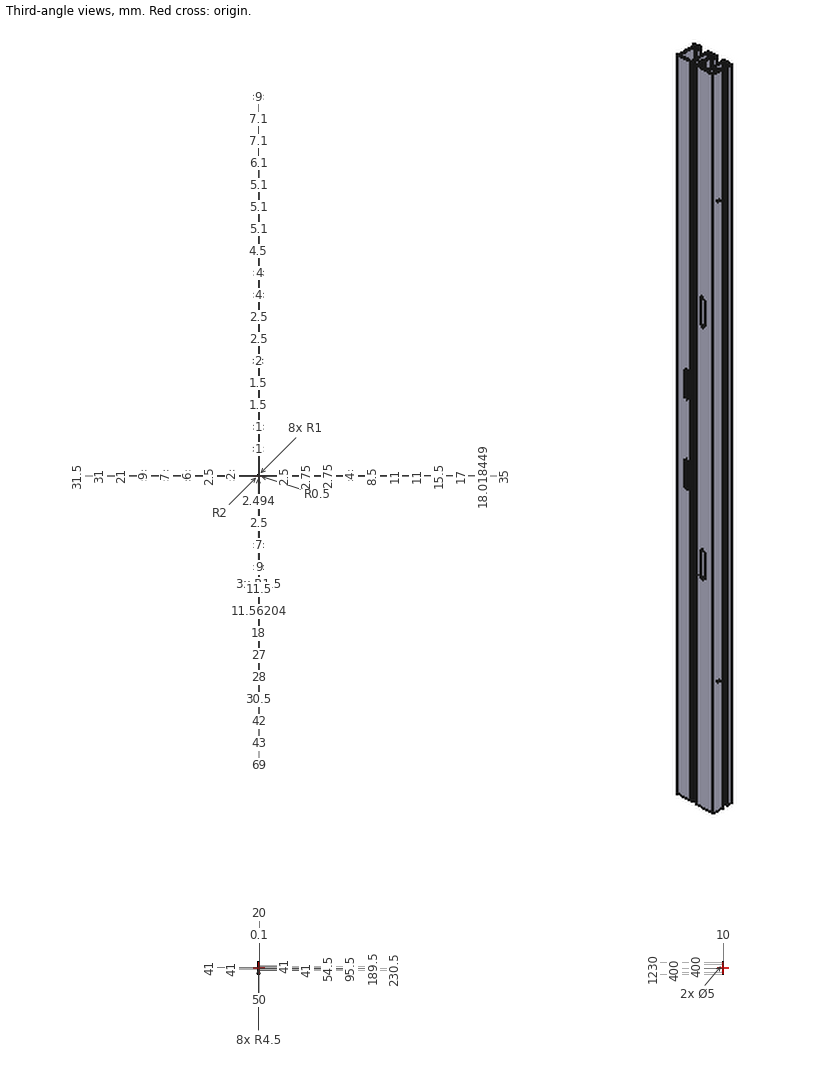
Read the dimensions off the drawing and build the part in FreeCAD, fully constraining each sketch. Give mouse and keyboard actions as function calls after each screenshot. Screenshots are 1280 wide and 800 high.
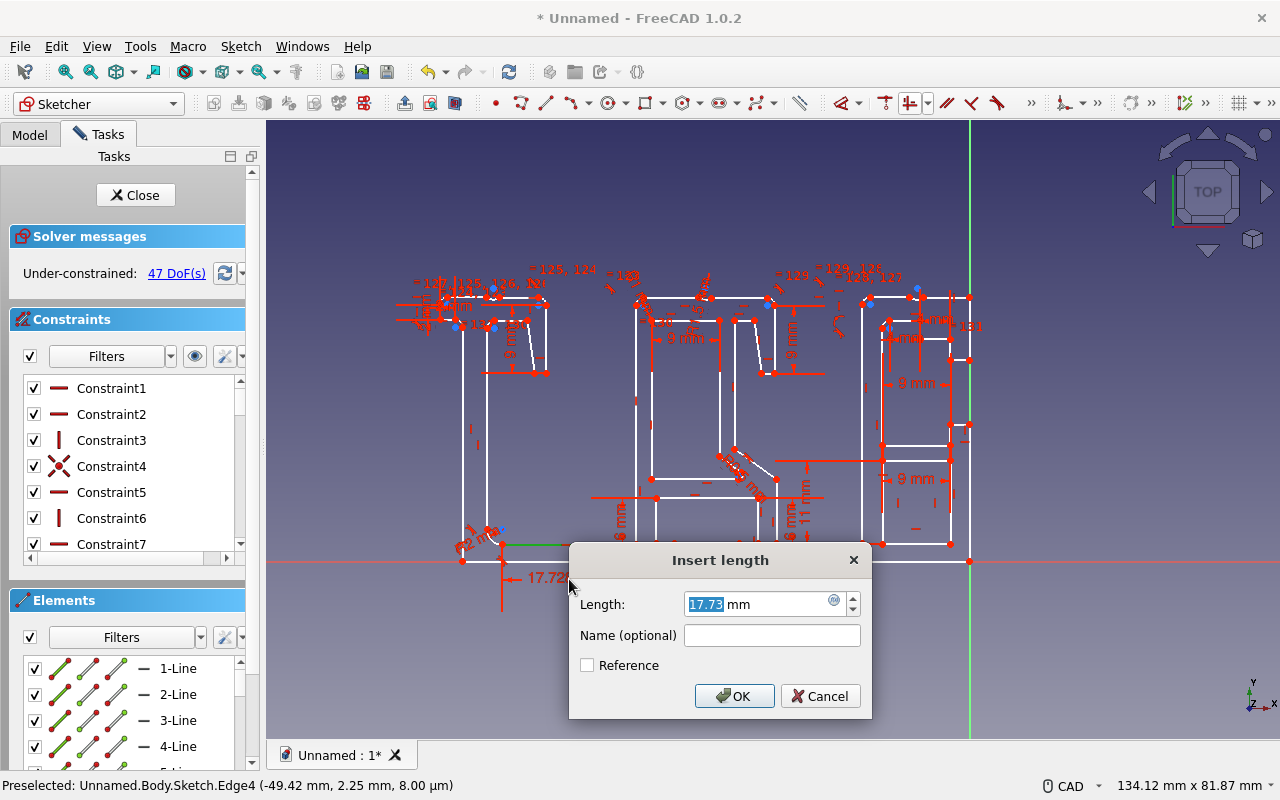
text(18)
key(Return)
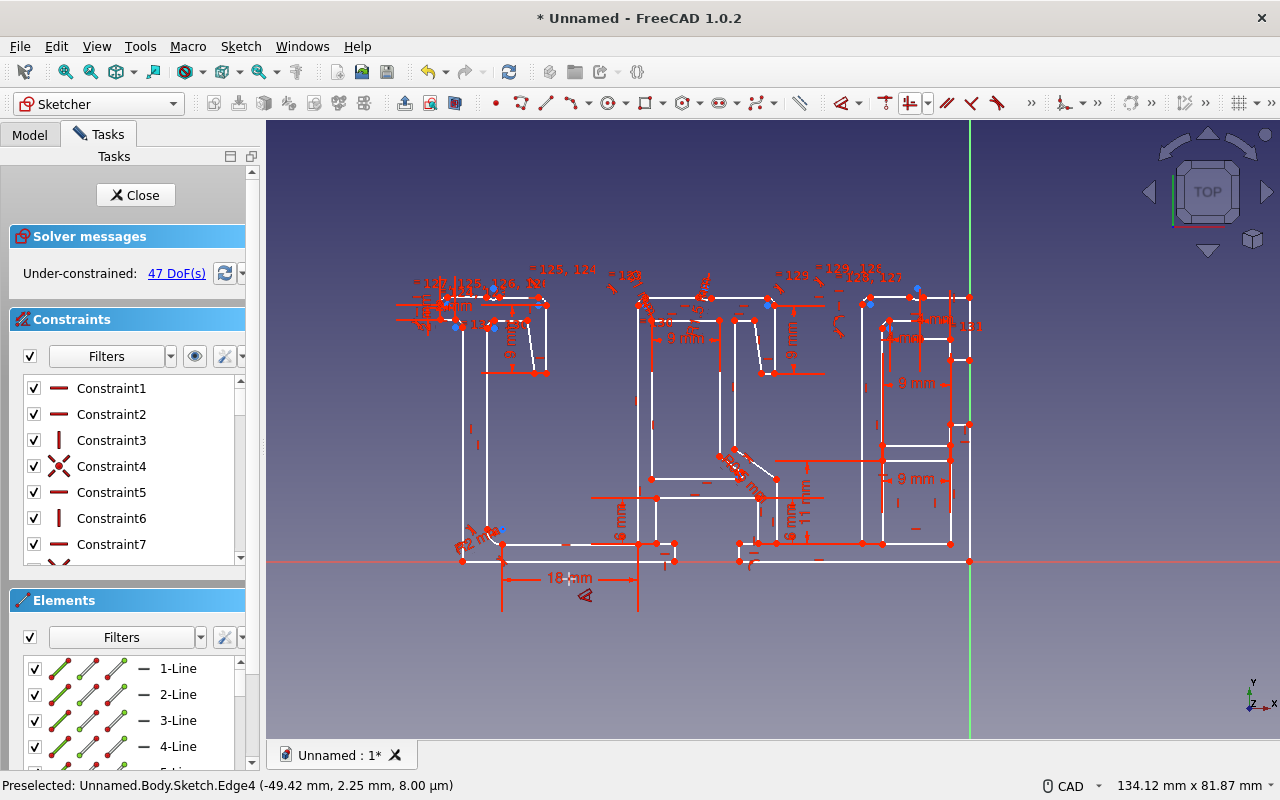
click(463, 398)
click(429, 445)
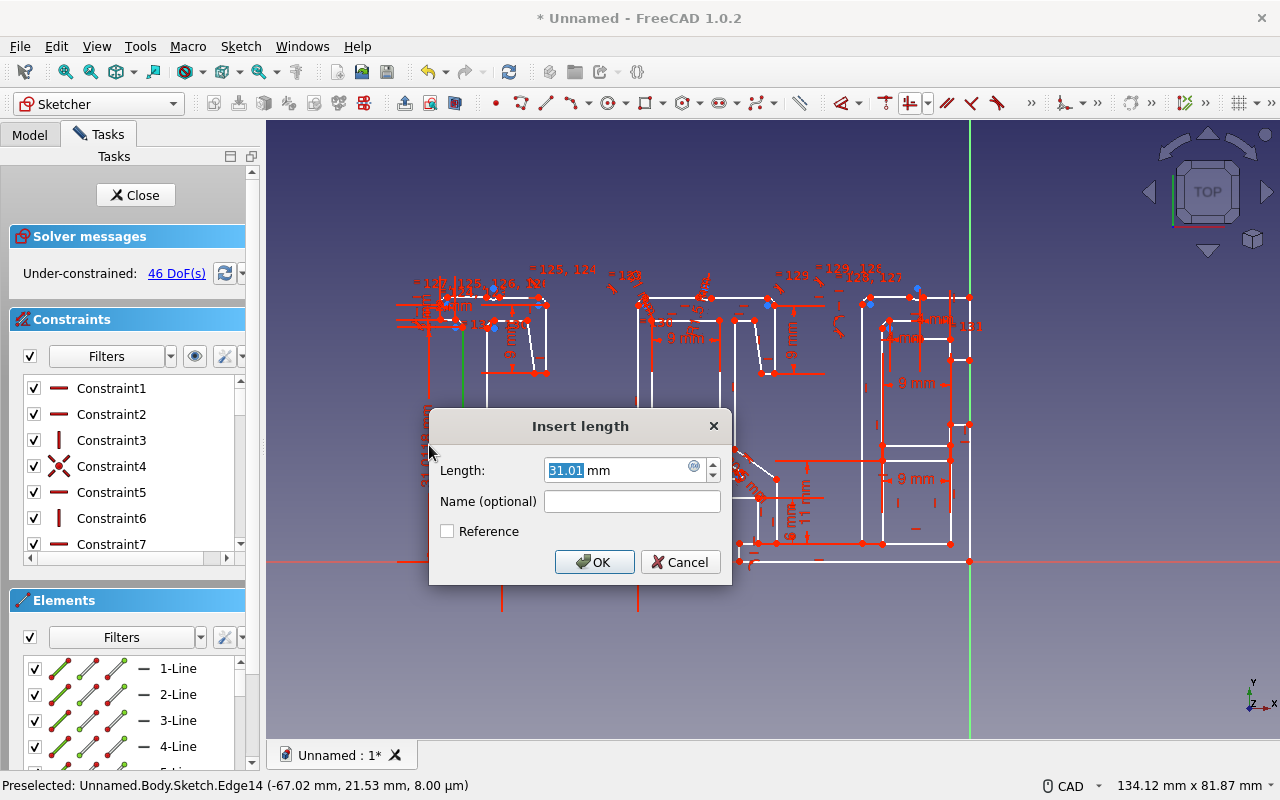
text(31)
key(Return)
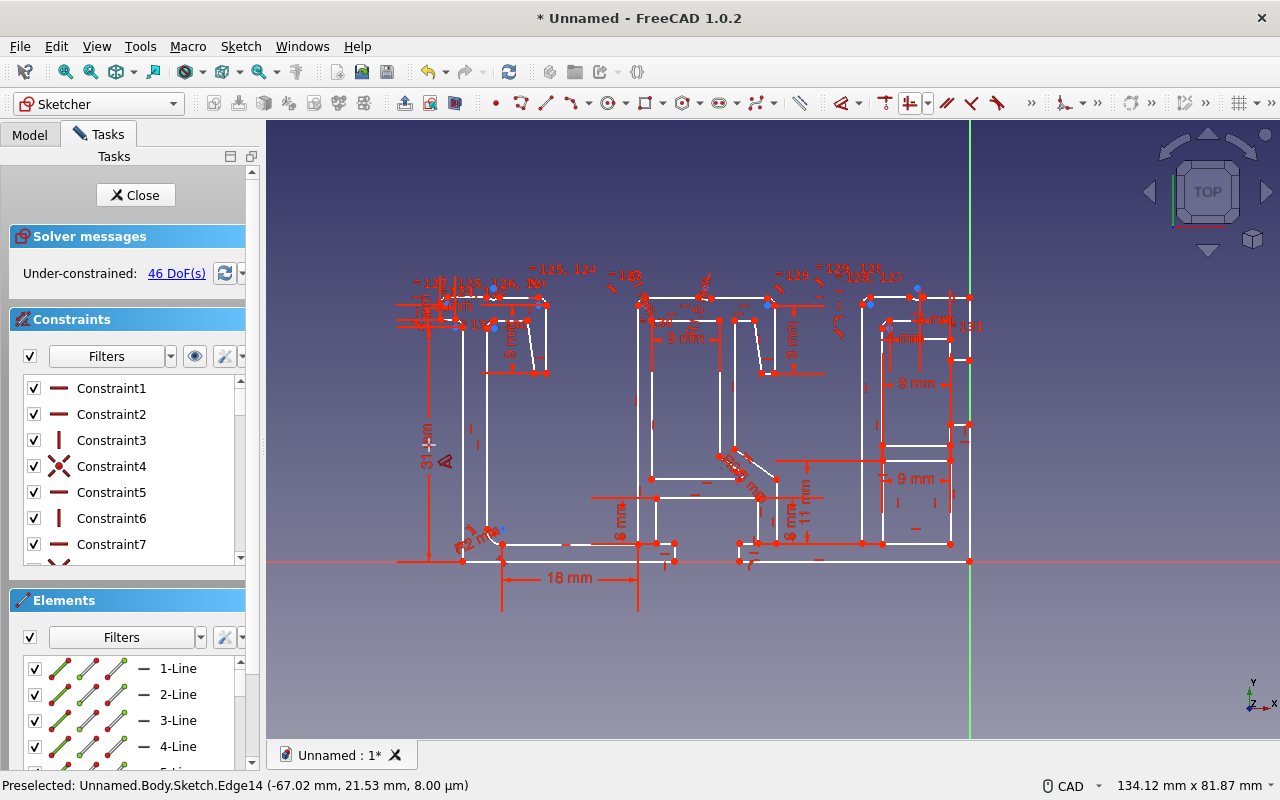
click(526, 562)
click(495, 596)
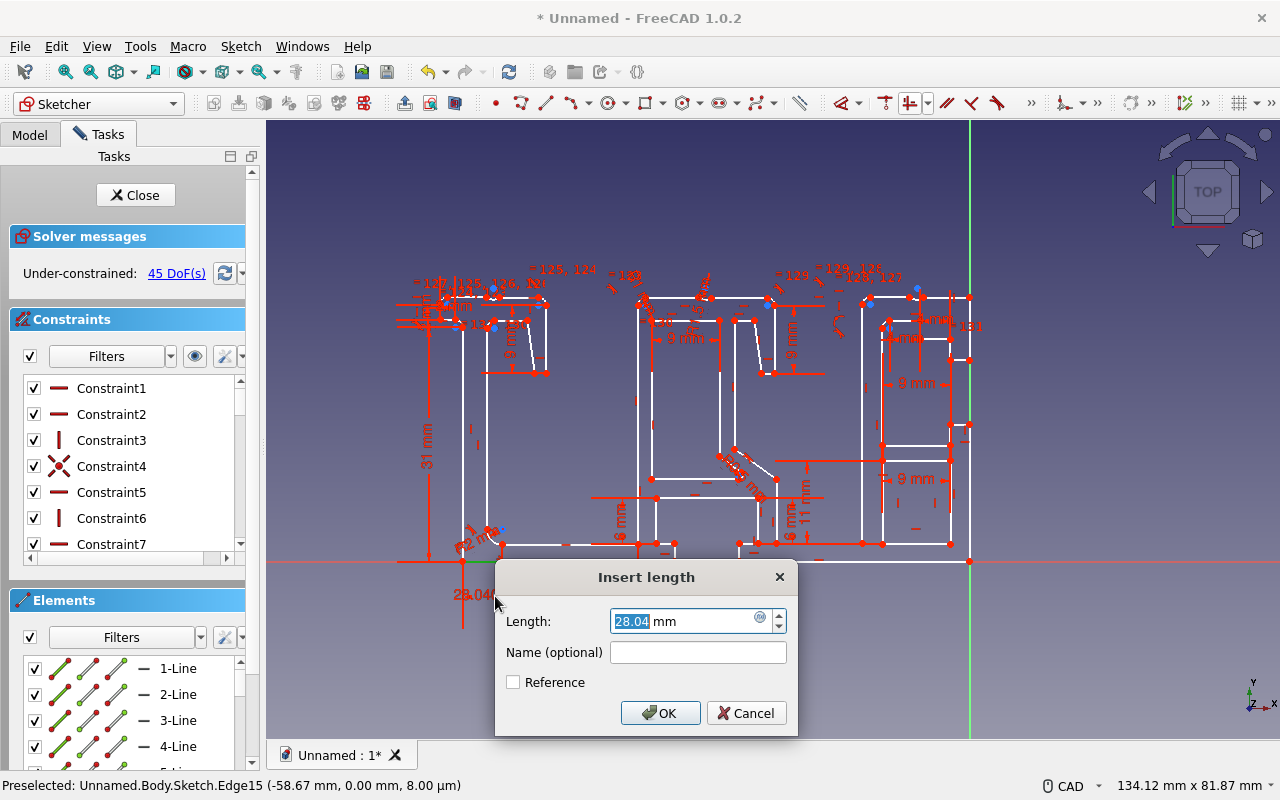
text(28)
key(Return)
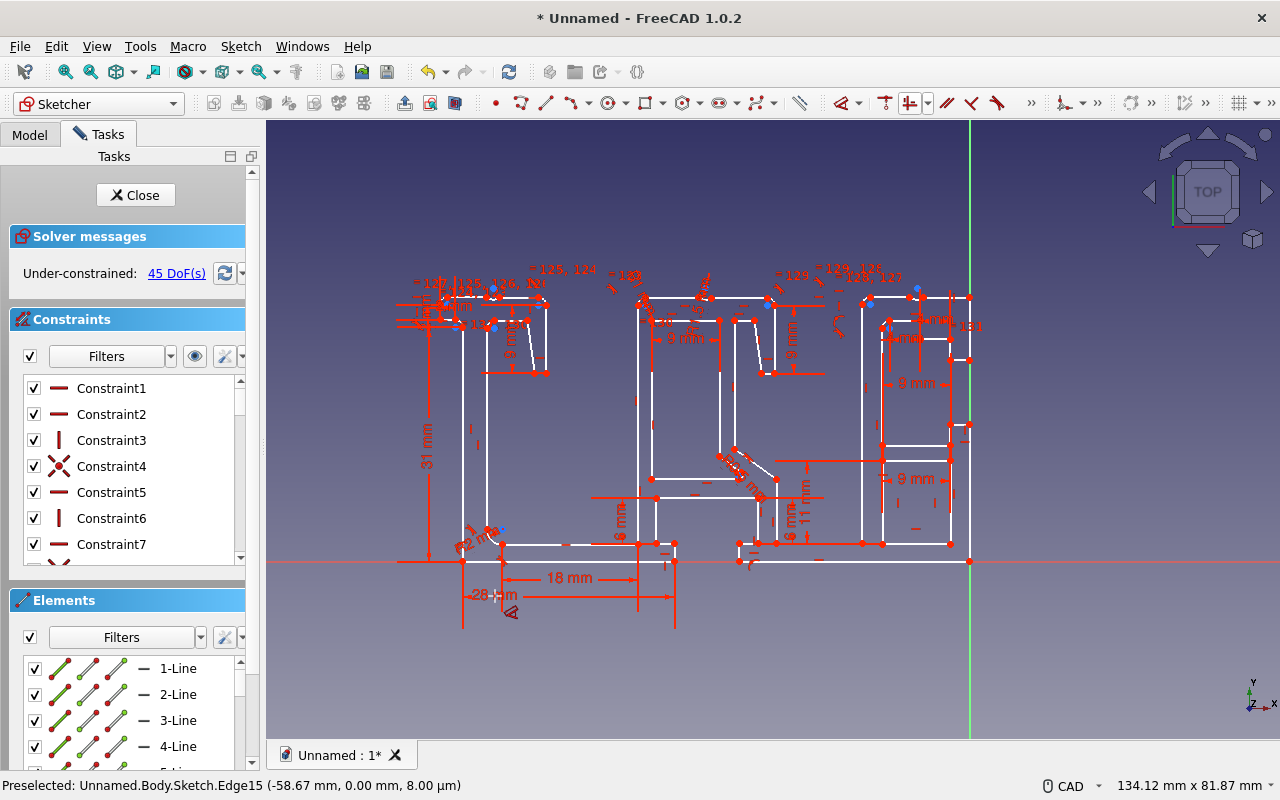
click(735, 411)
click(769, 414)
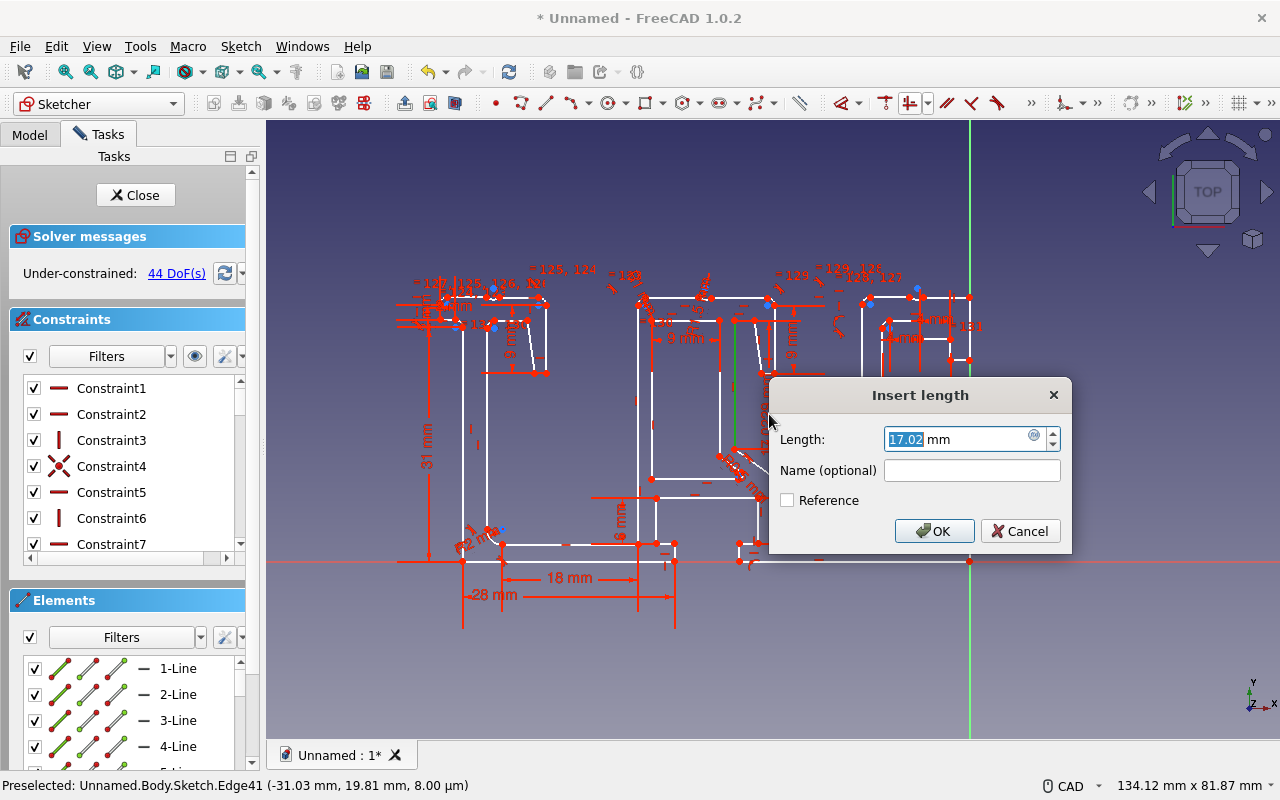
text(17)
key(Return)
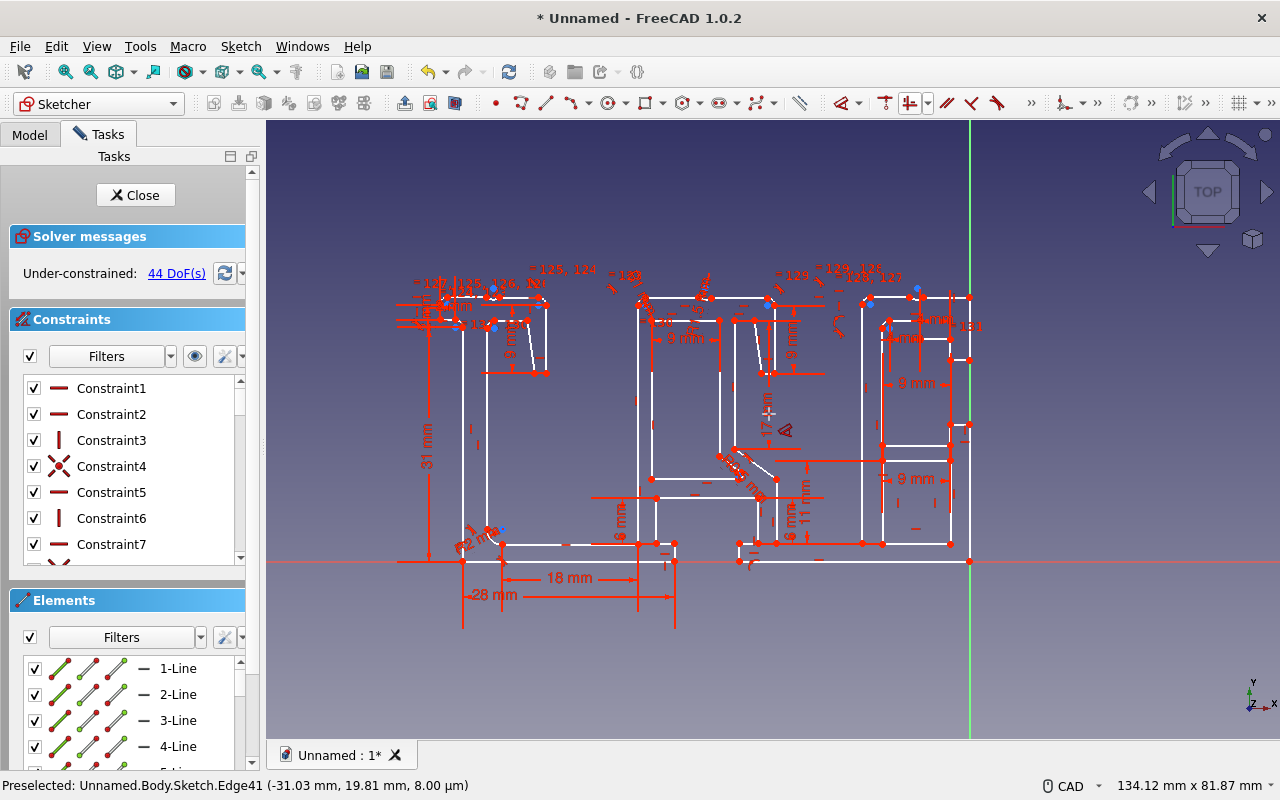
click(652, 432)
click(618, 400)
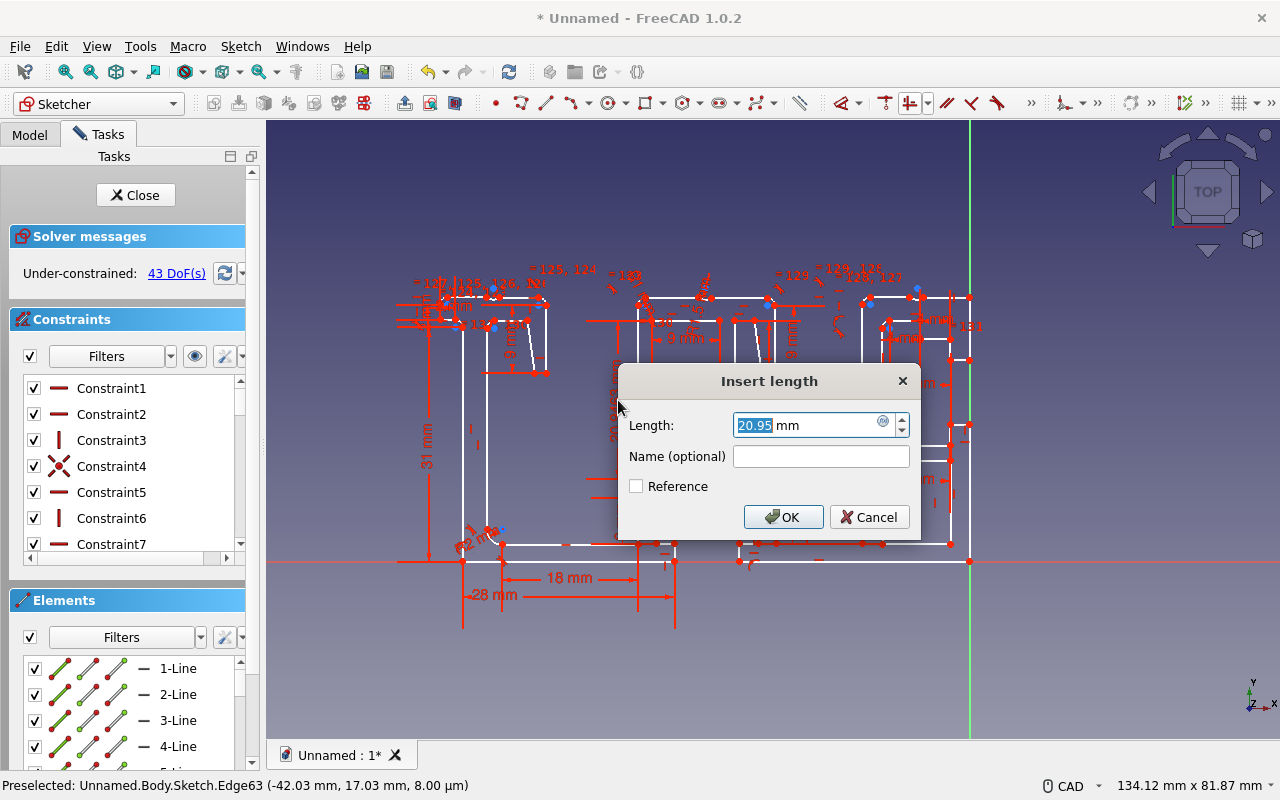
text(21)
key(Return)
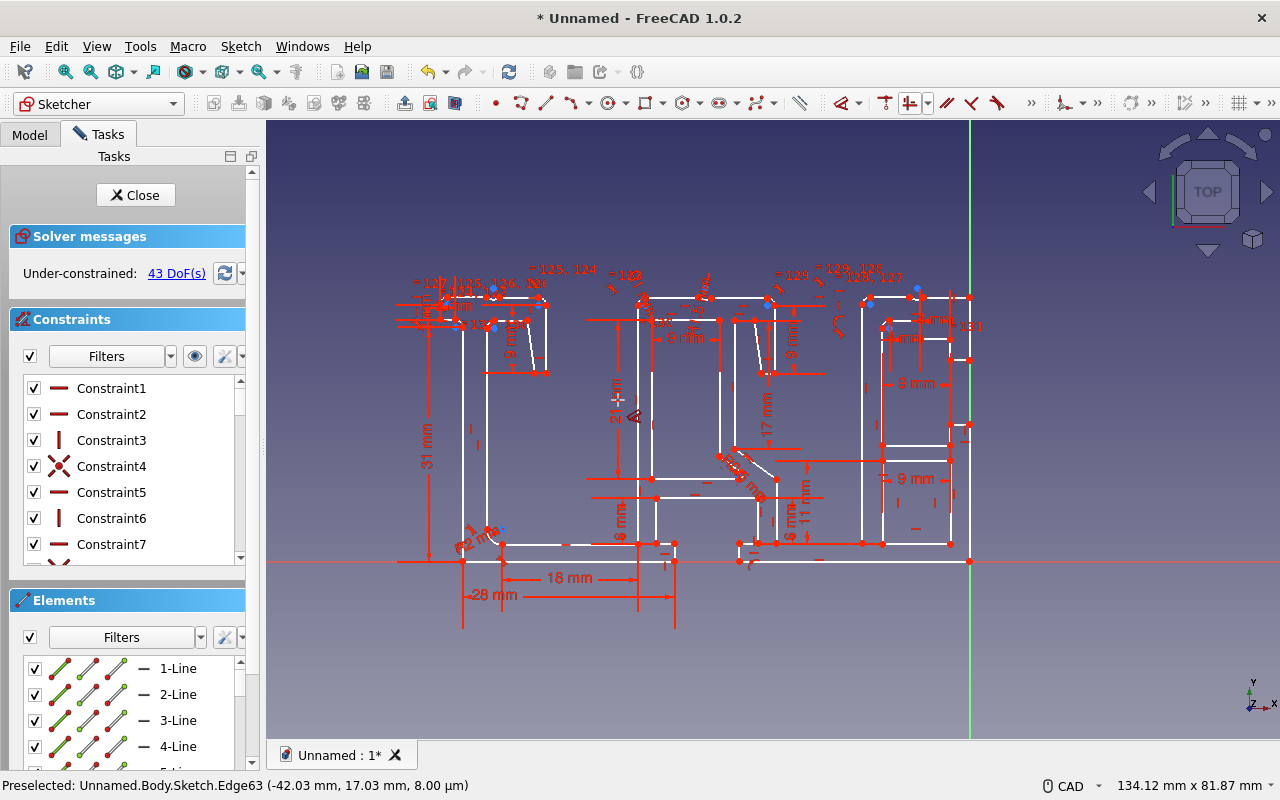
scroll(530, 336, up, 9)